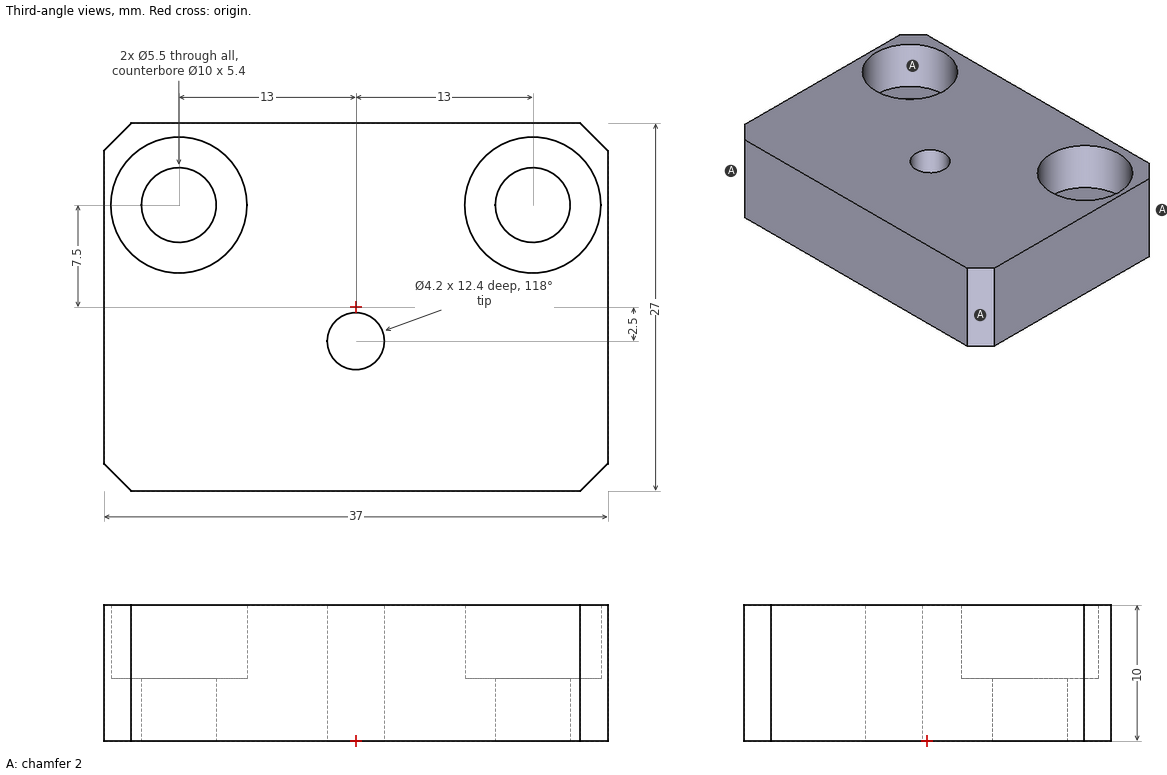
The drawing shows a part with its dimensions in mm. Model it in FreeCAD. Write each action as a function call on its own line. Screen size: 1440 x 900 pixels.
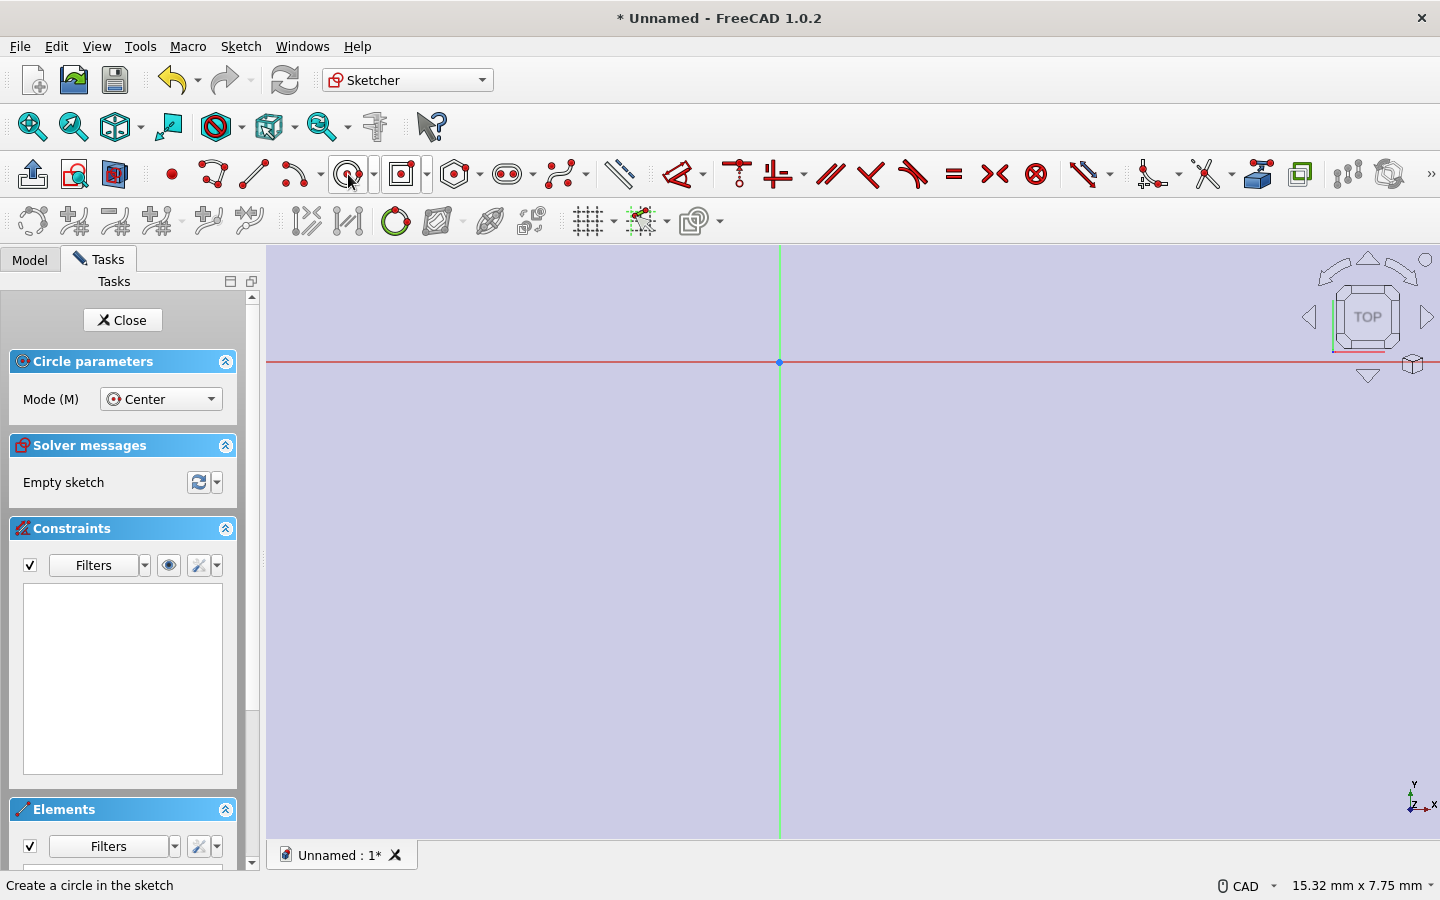
click(780, 554)
move(894, 440)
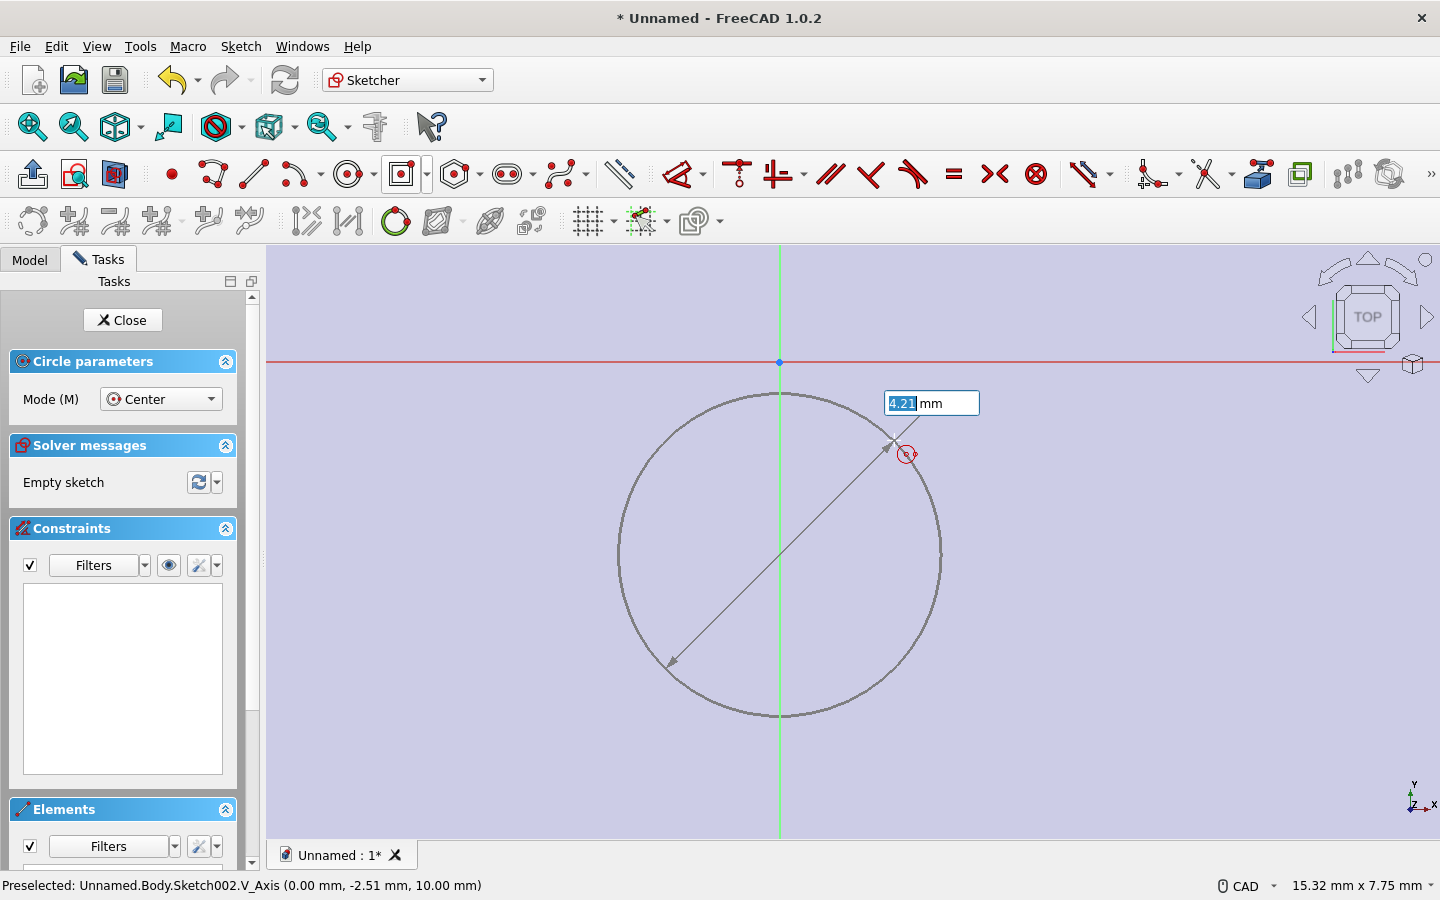
text(4.2)
key(Return)
key(Escape)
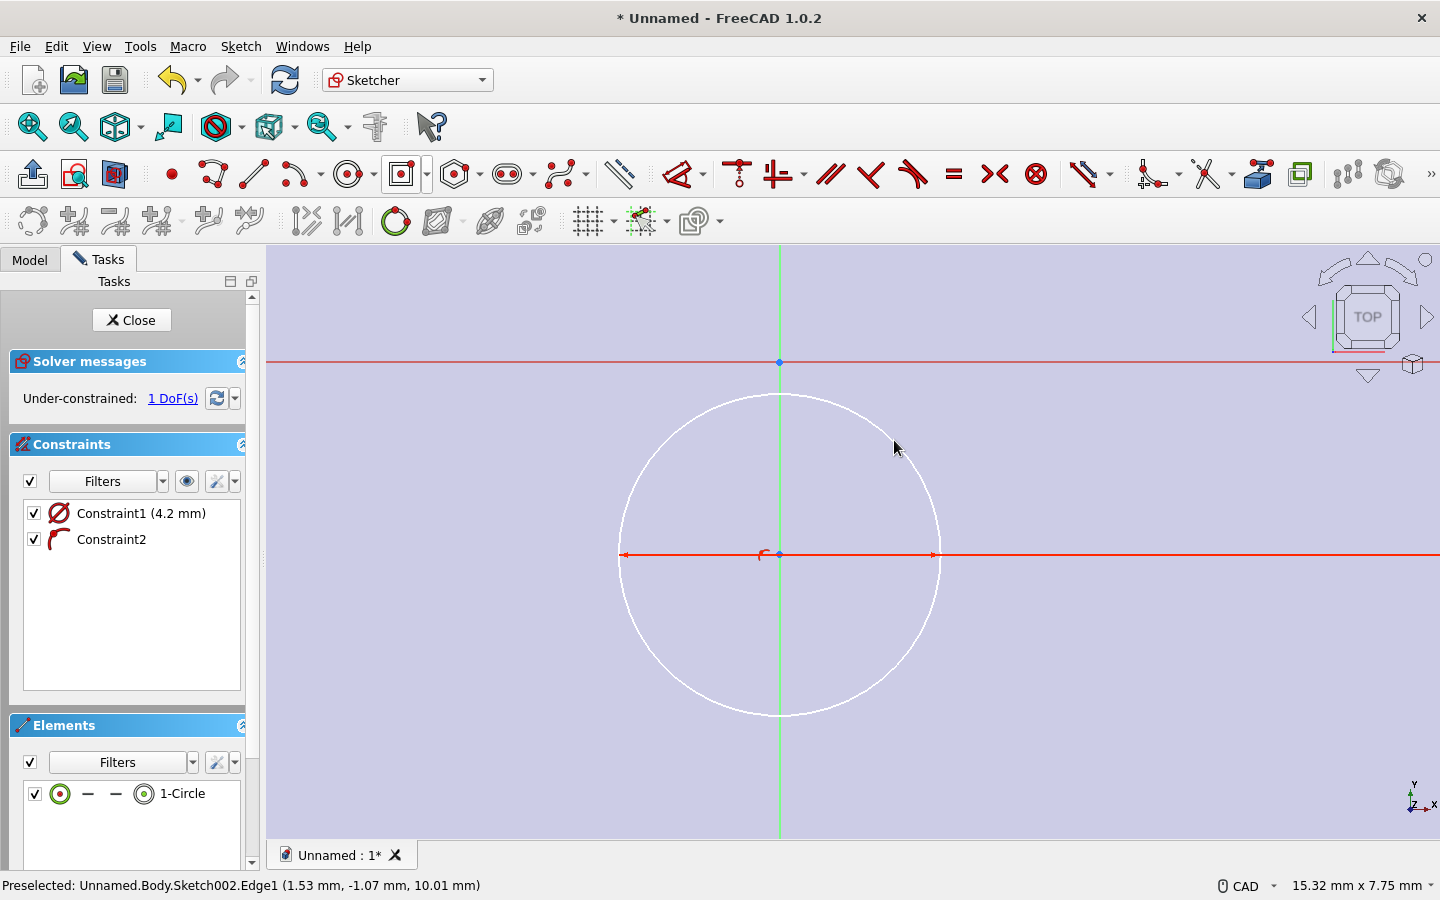
click(676, 174)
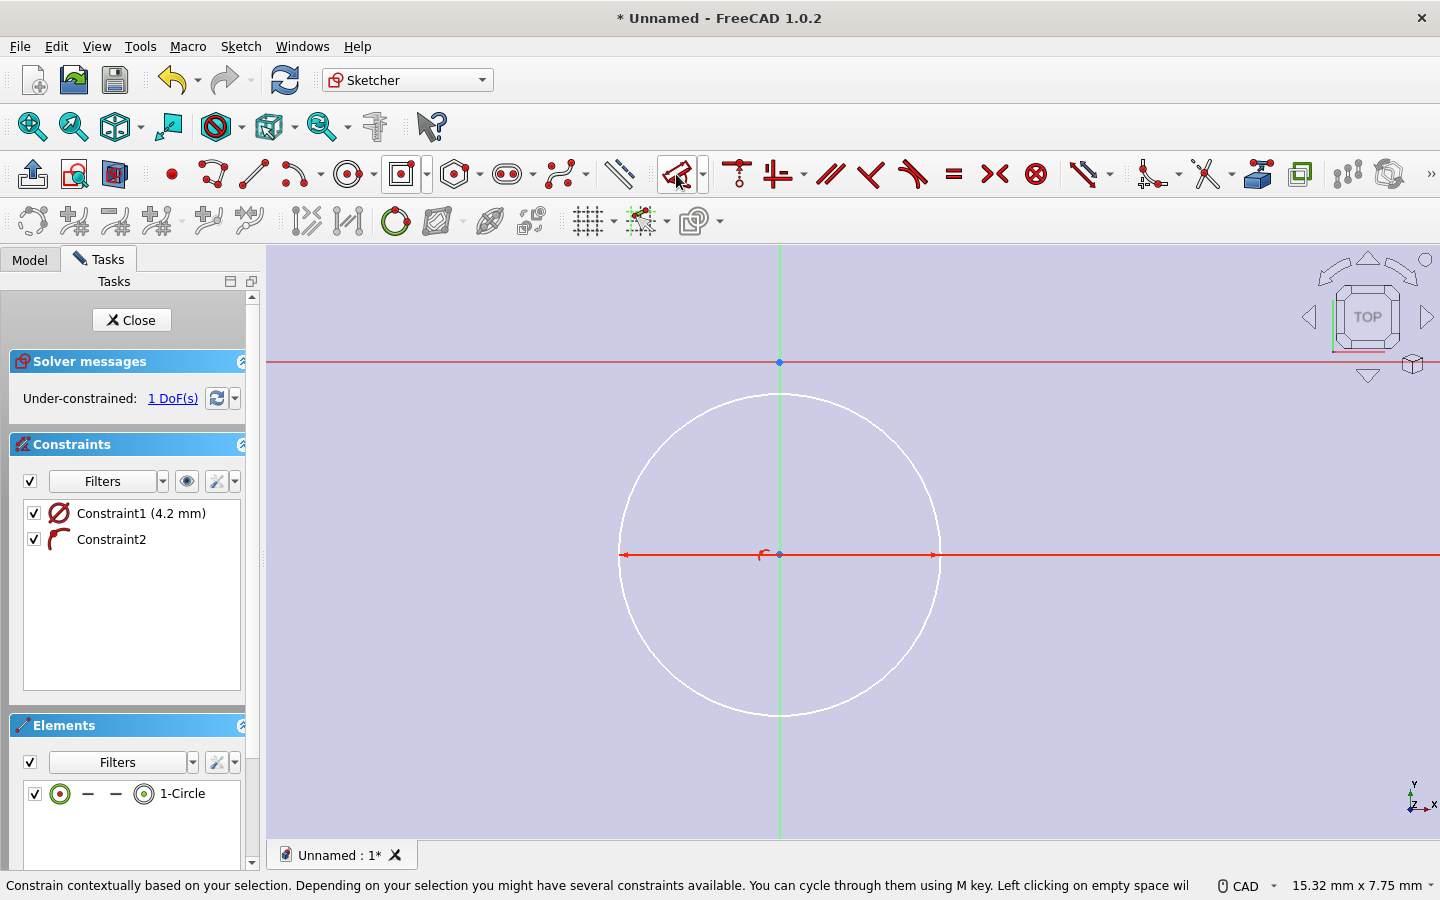
click(780, 555)
click(814, 459)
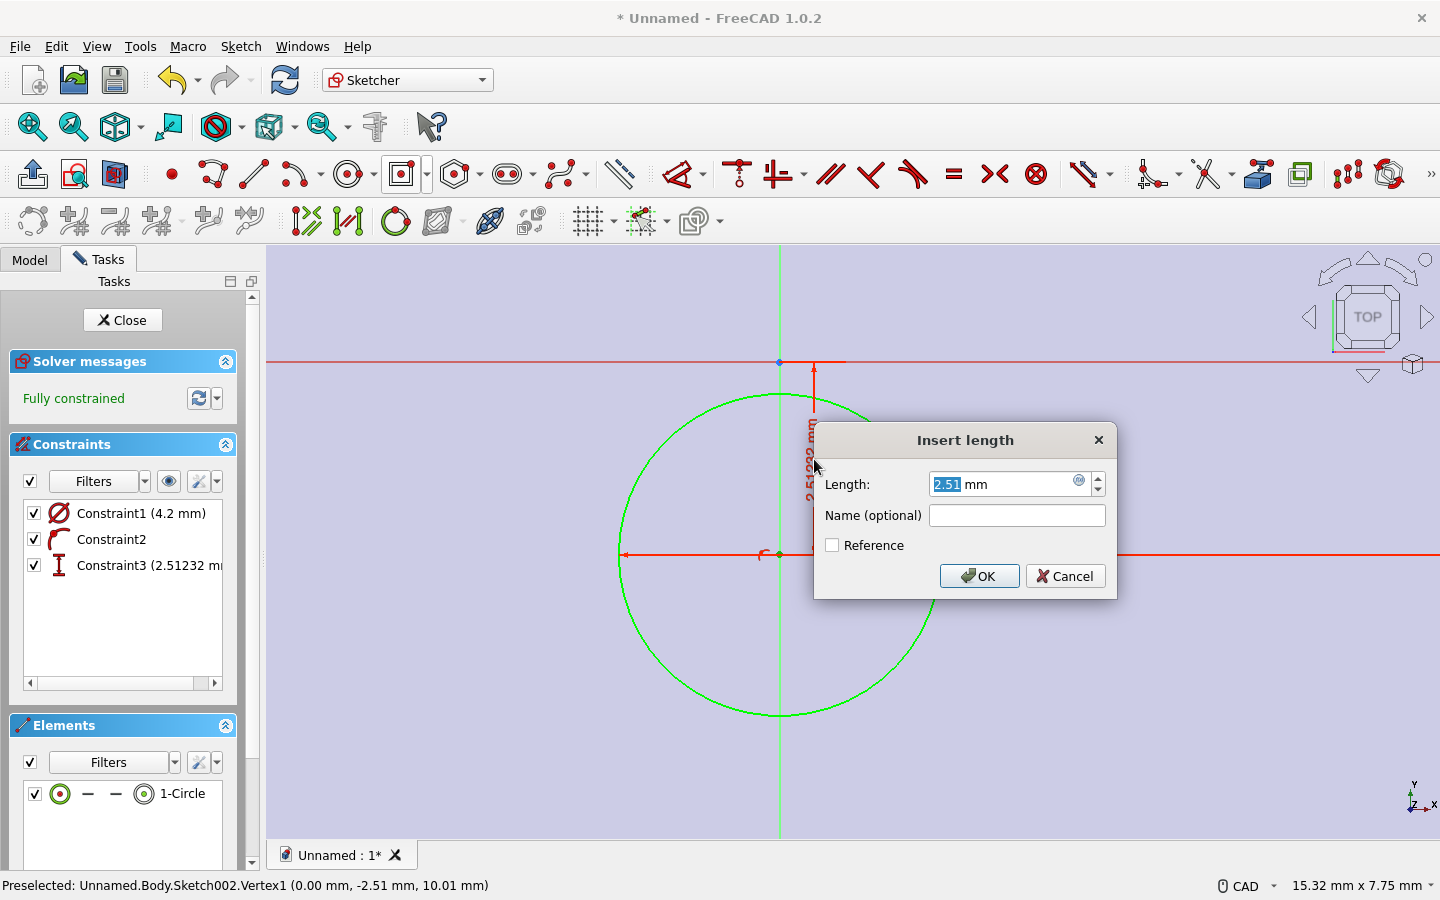
text(2.5)
key(Return)
key(Escape)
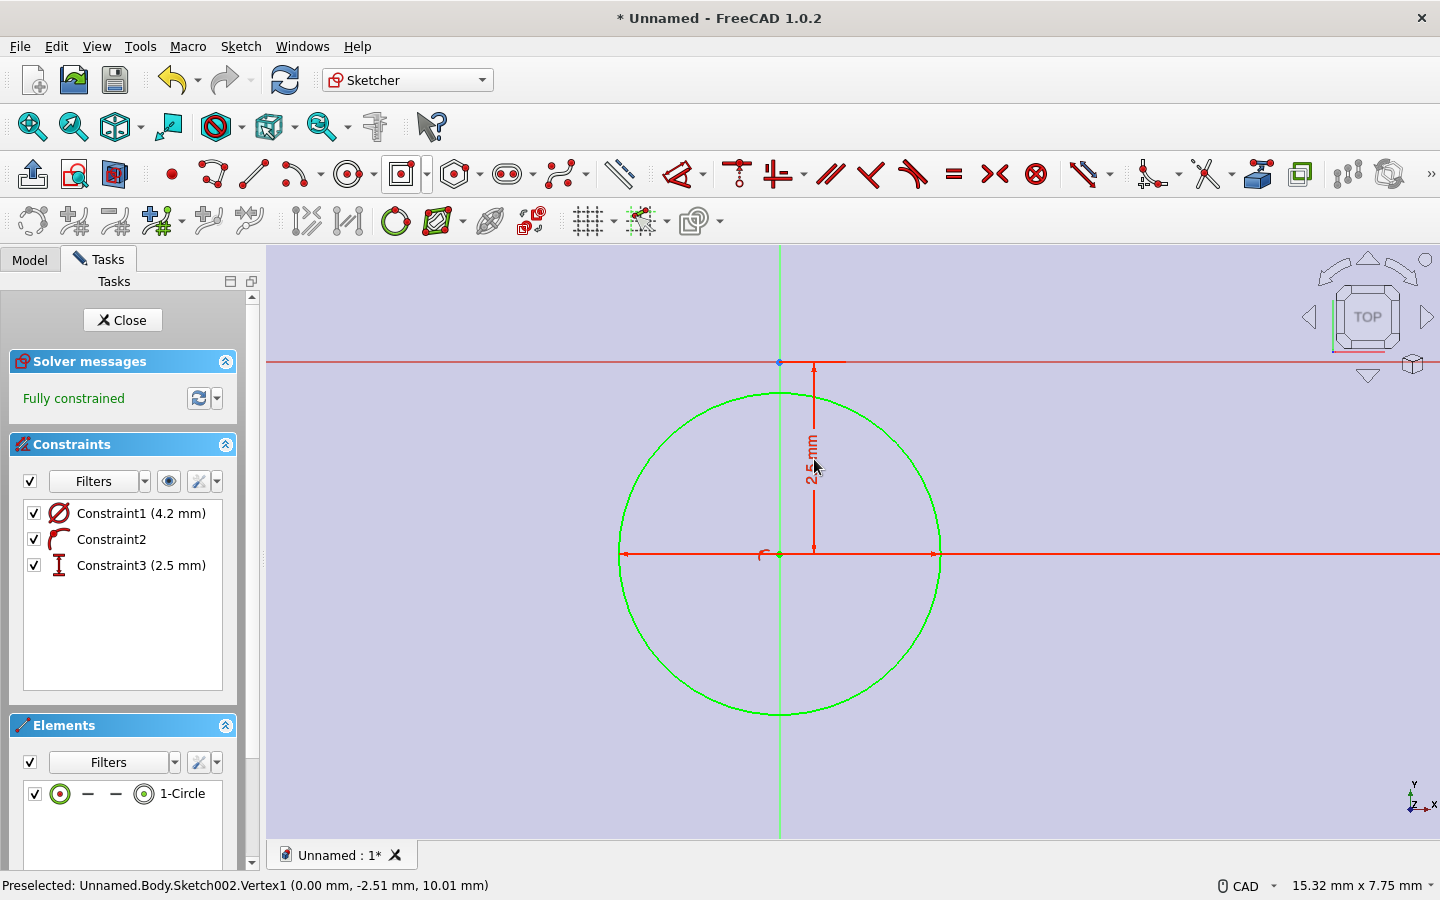
click(123, 320)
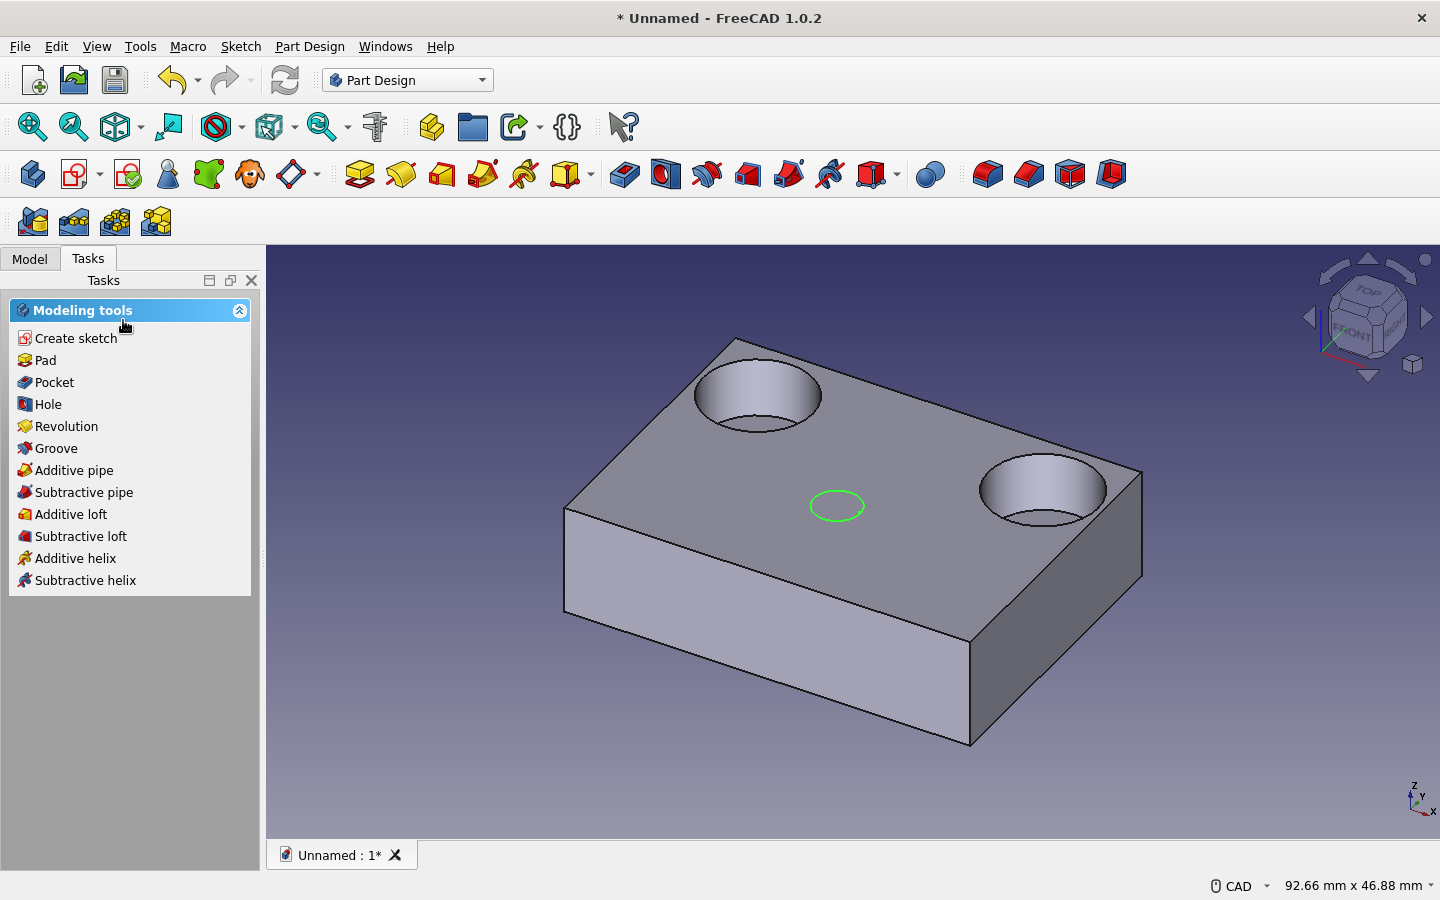
click(666, 174)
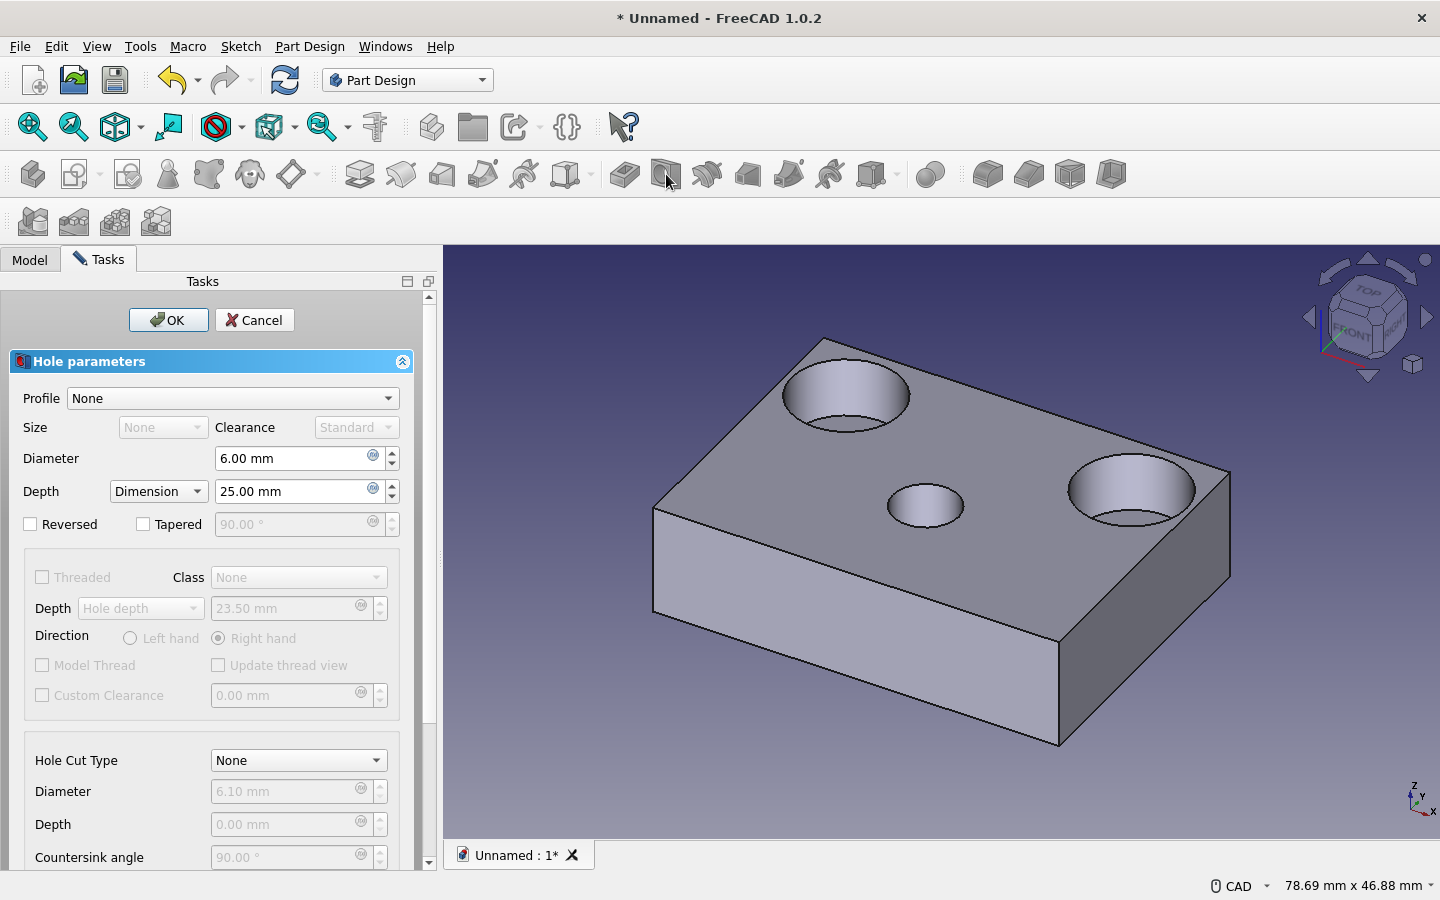
triple_click(300, 458)